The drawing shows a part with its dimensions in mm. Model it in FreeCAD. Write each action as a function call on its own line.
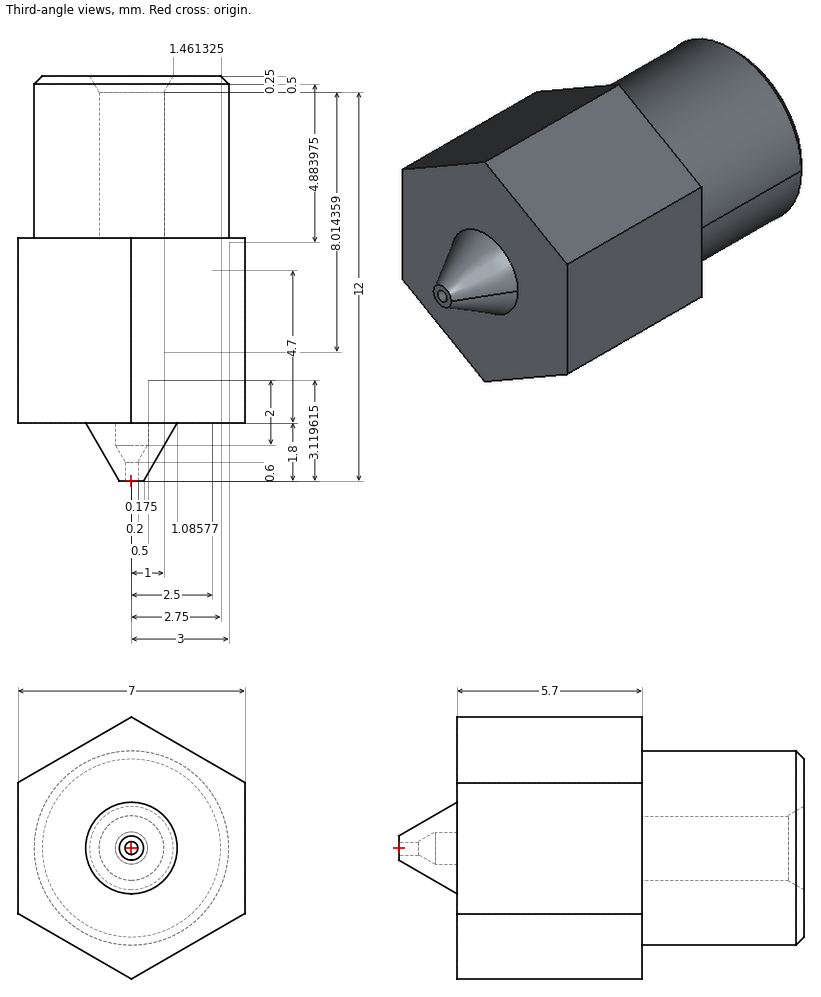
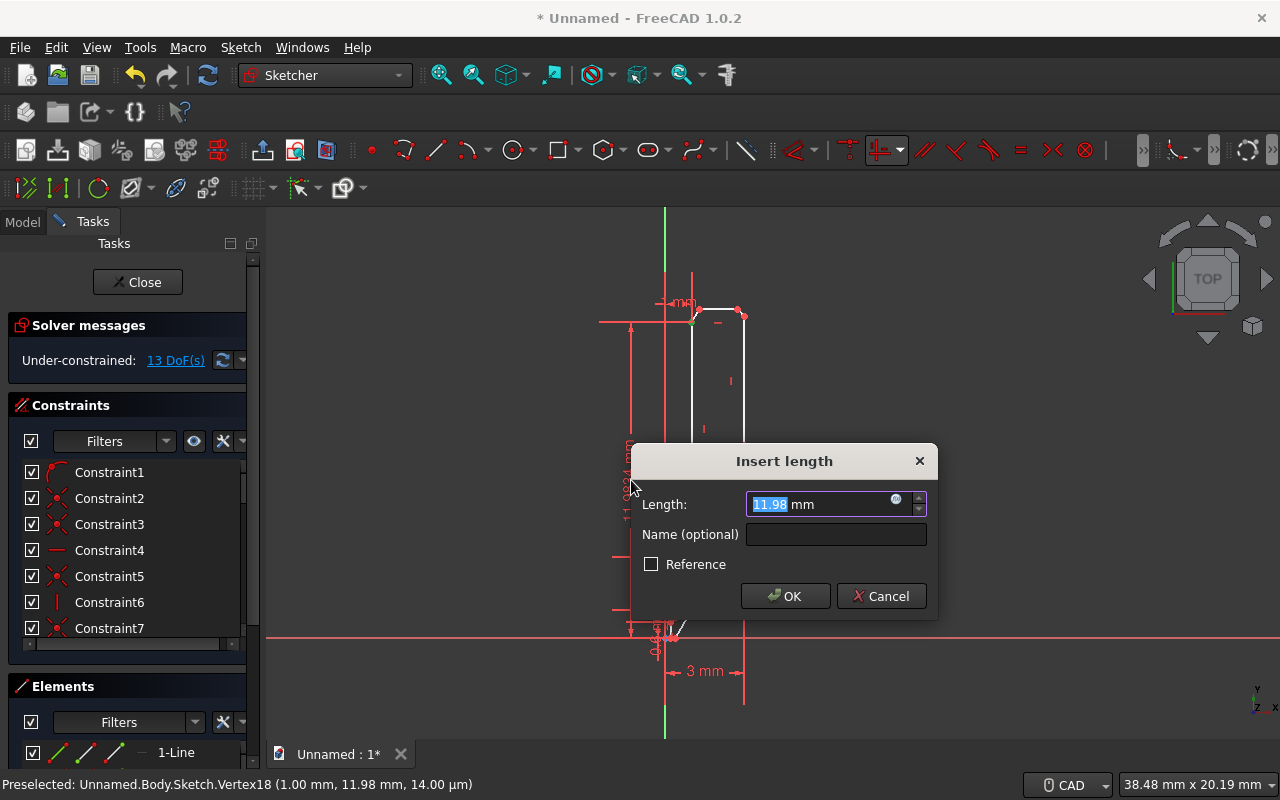
text(12)
key(Return)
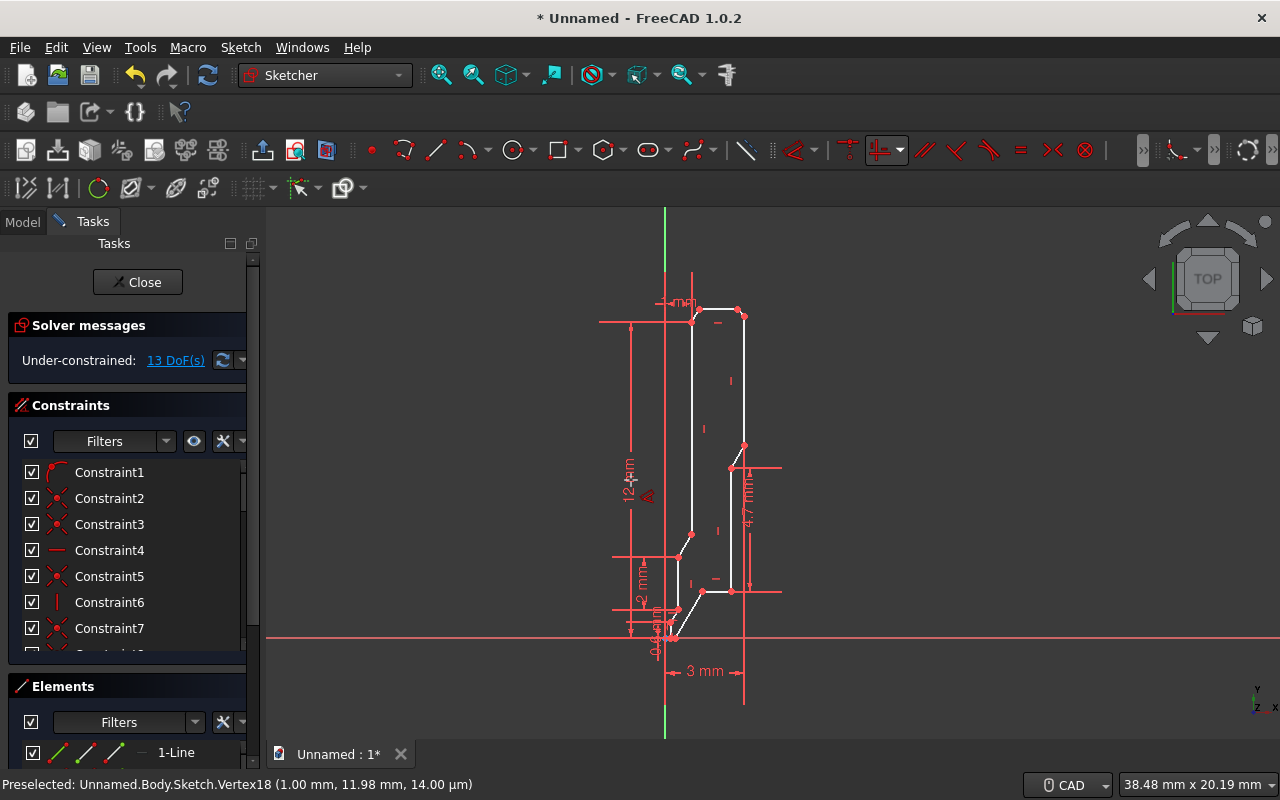
scroll(671, 638, up, 11)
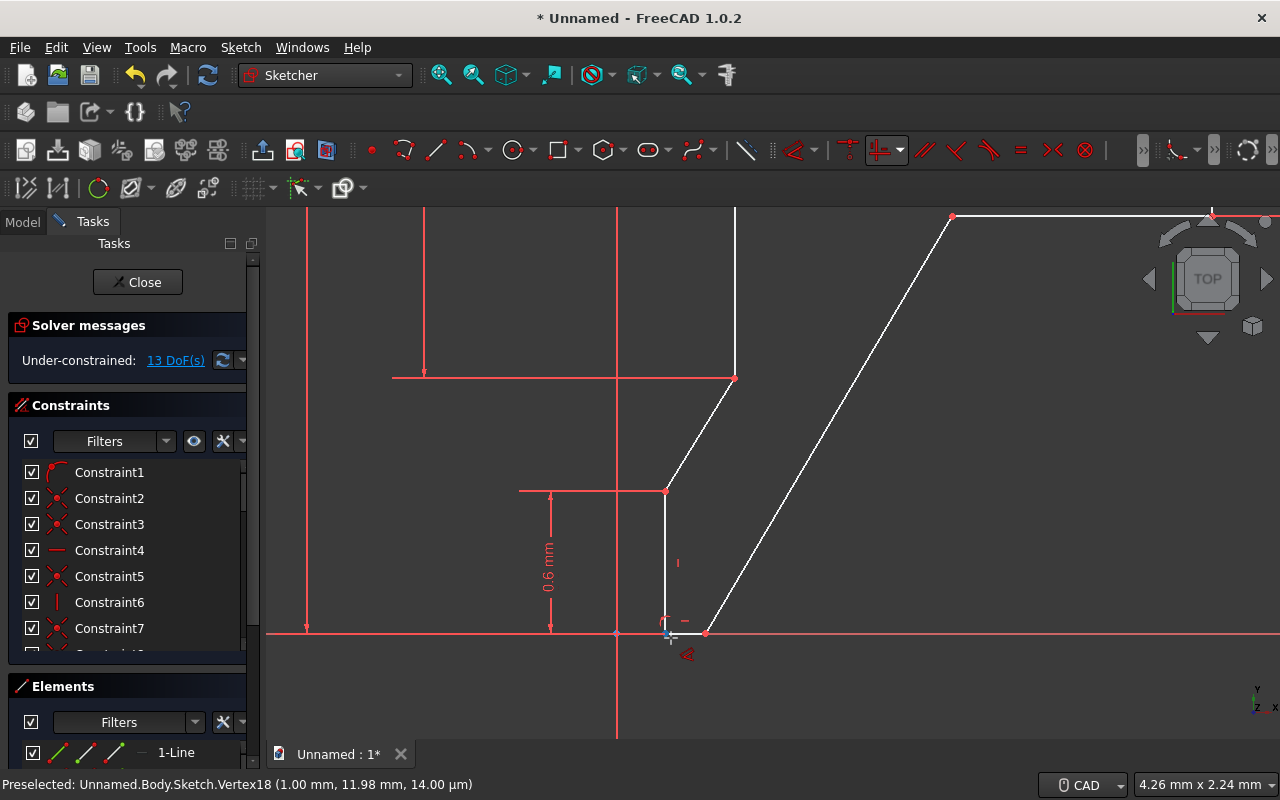
click(665, 634)
click(641, 668)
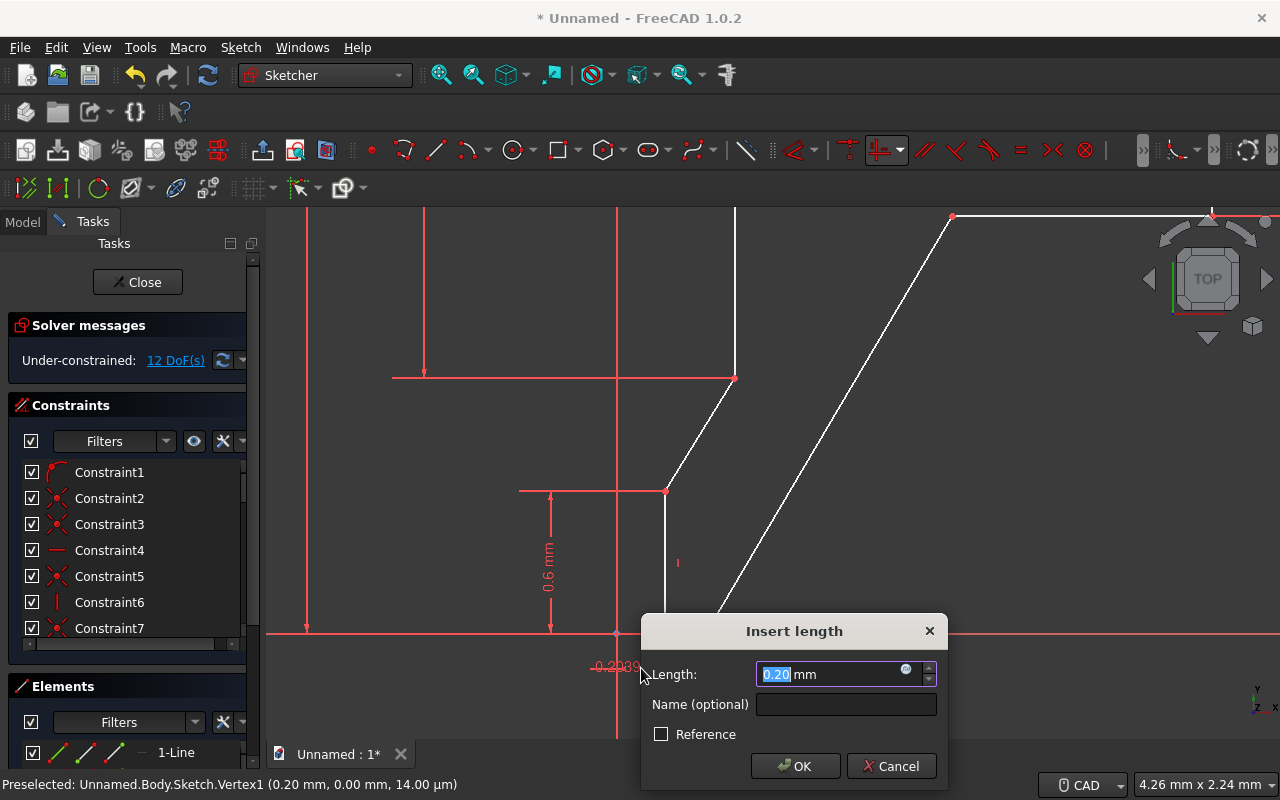
text(0.2)
key(Return)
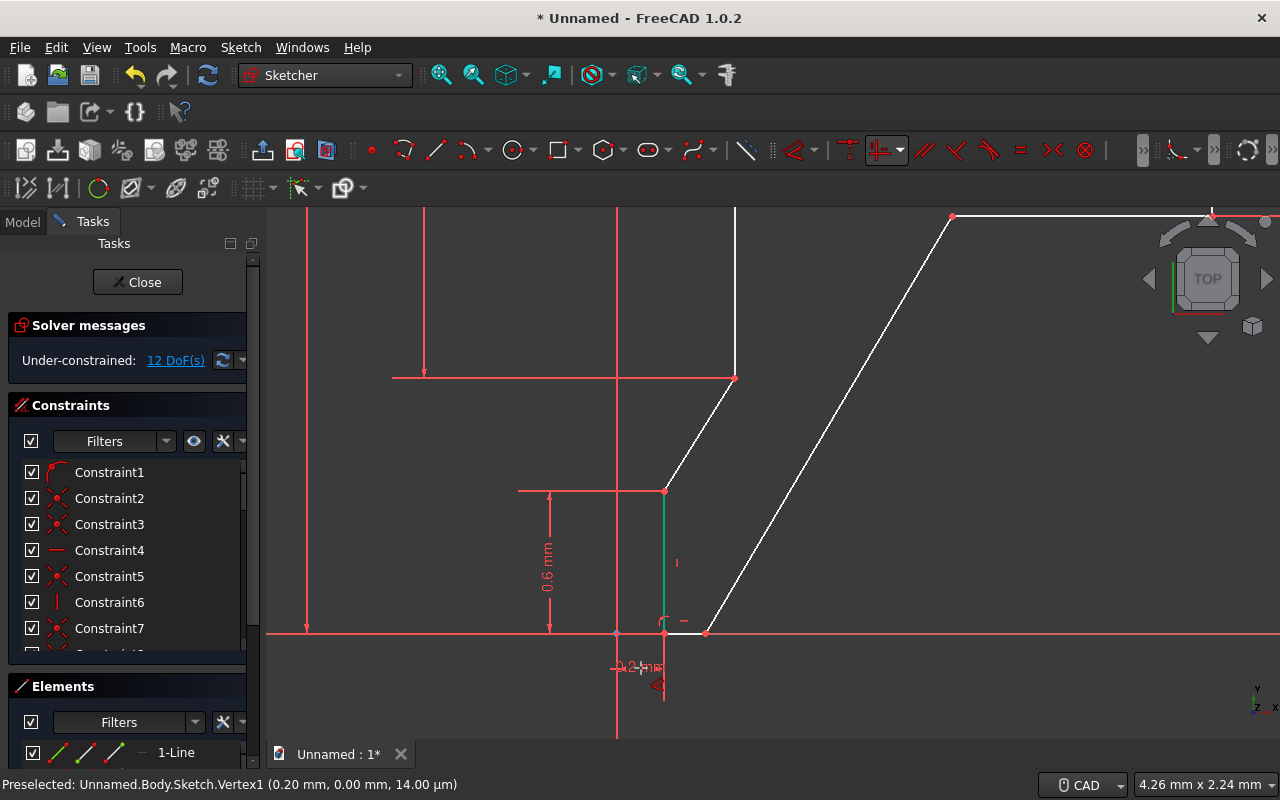
scroll(671, 638, down, 11)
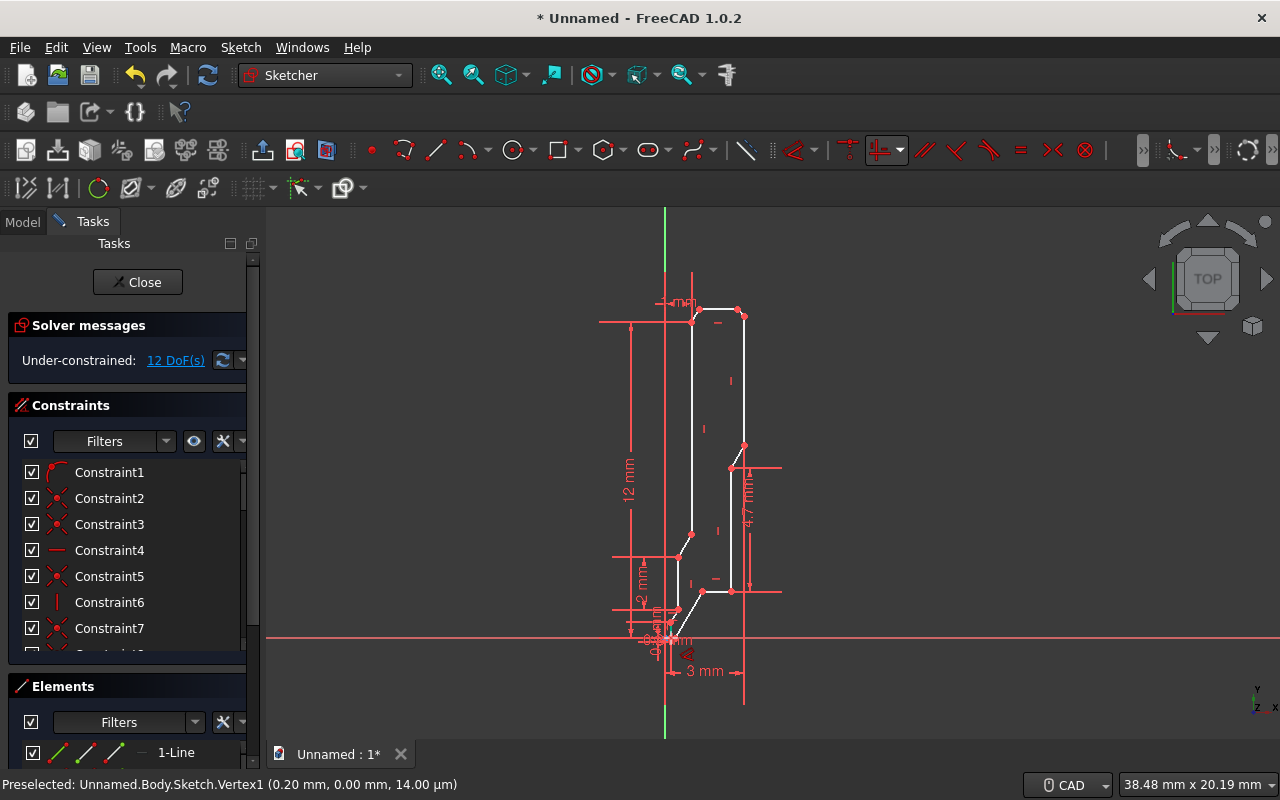
click(703, 592)
click(631, 604)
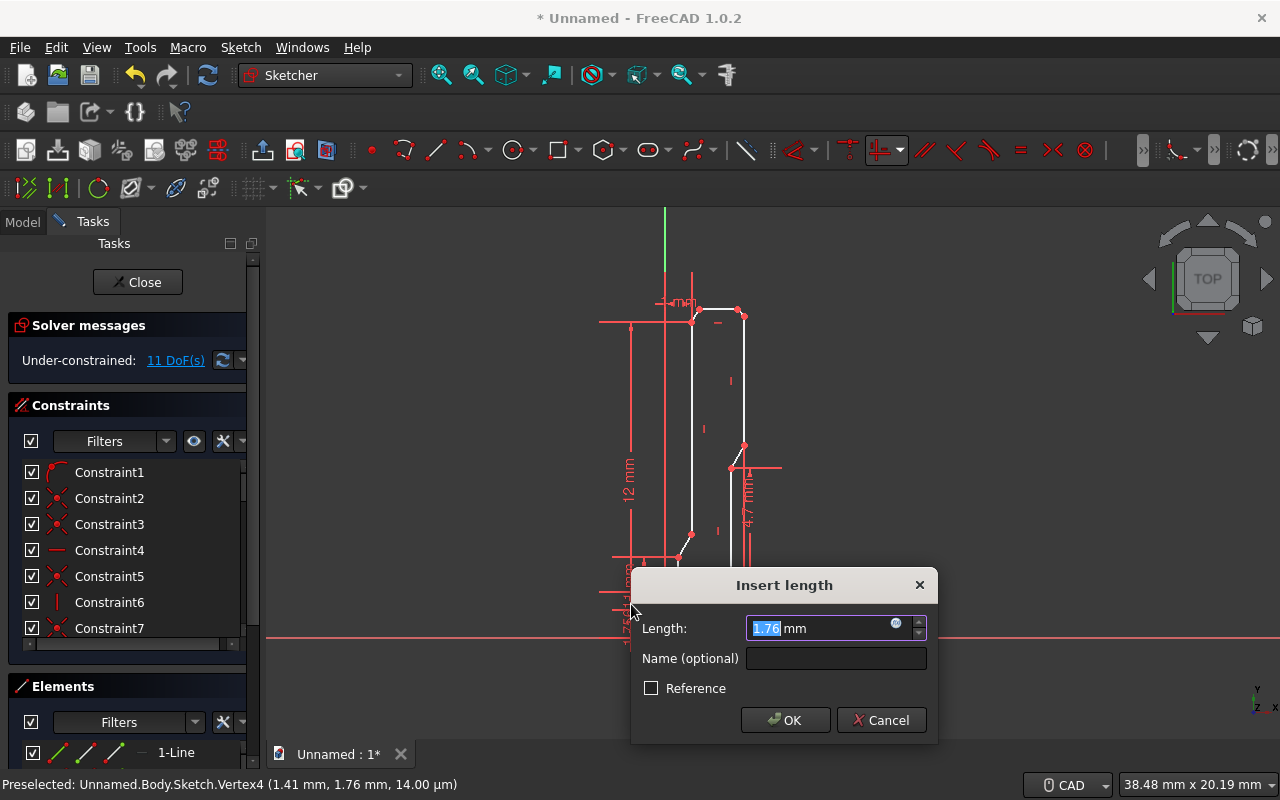
text(1.8)
key(Return)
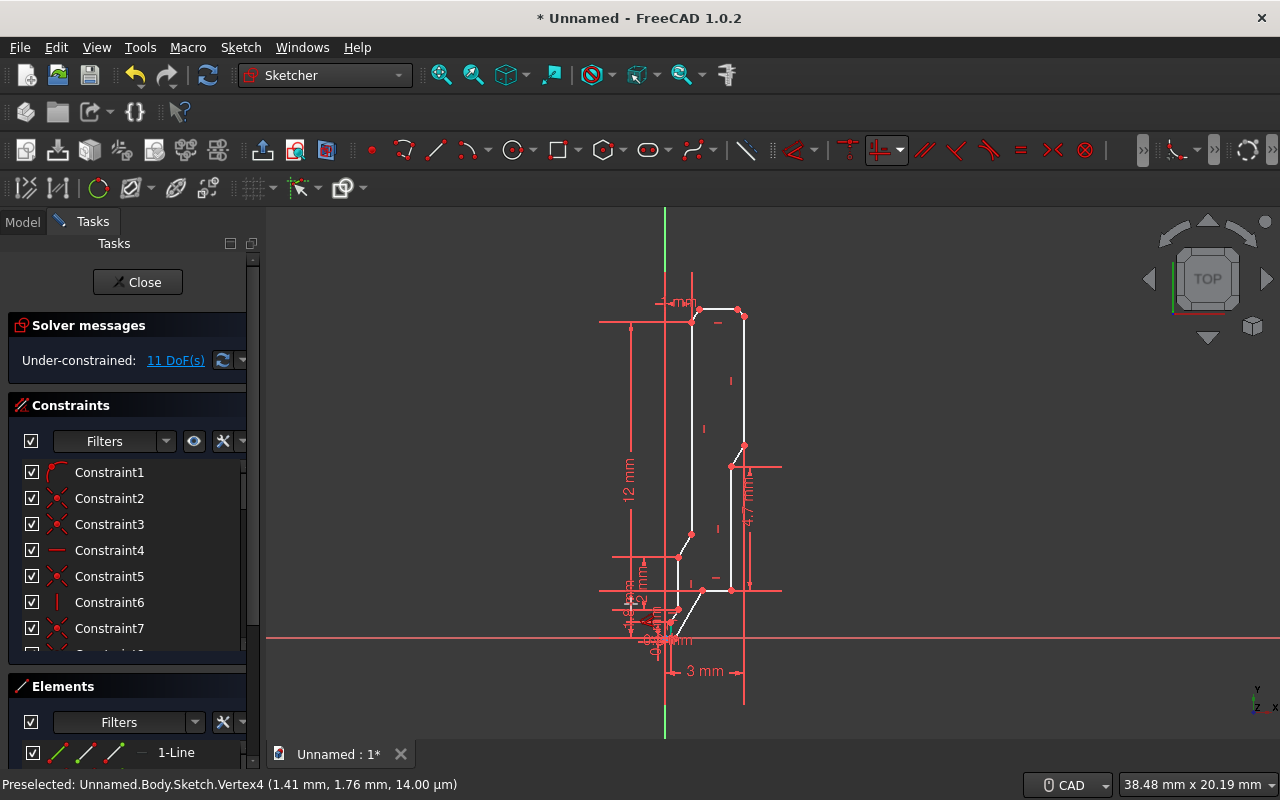
click(731, 591)
click(698, 557)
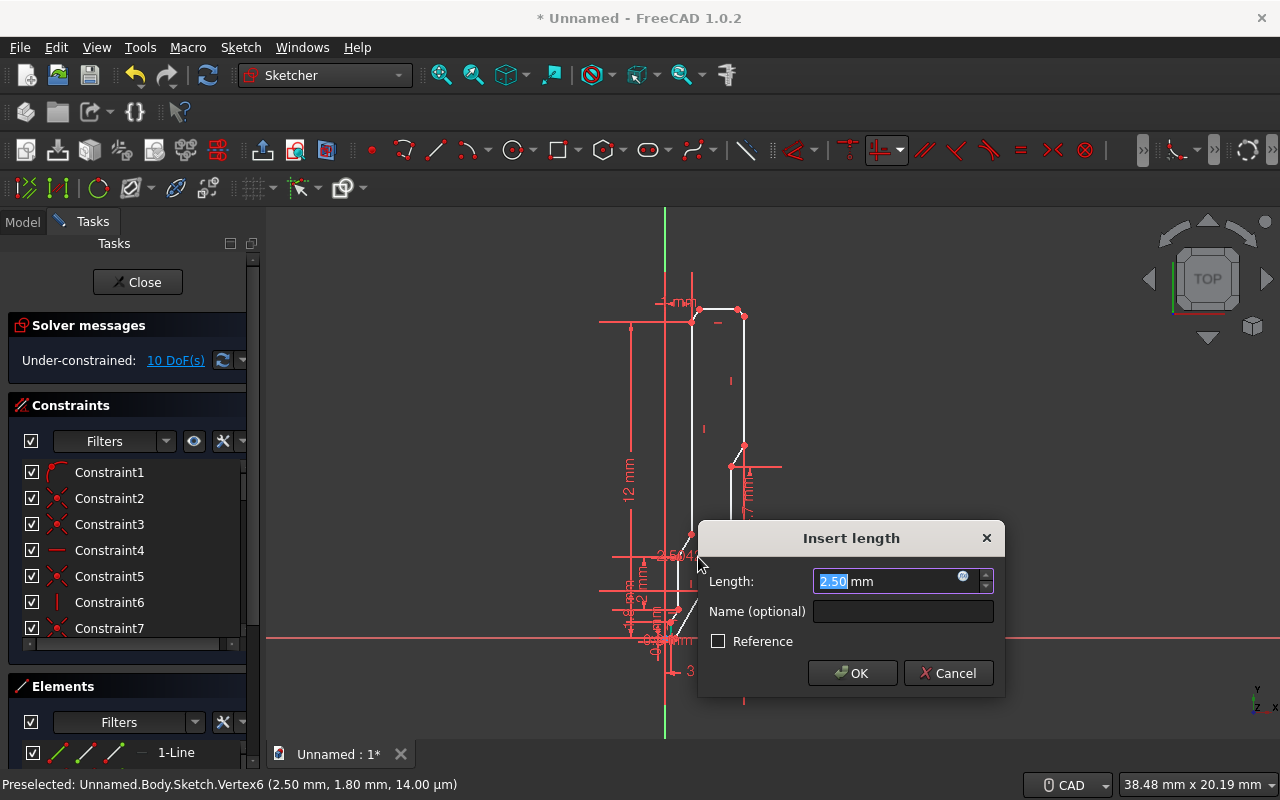
text(2.5)
key(Return)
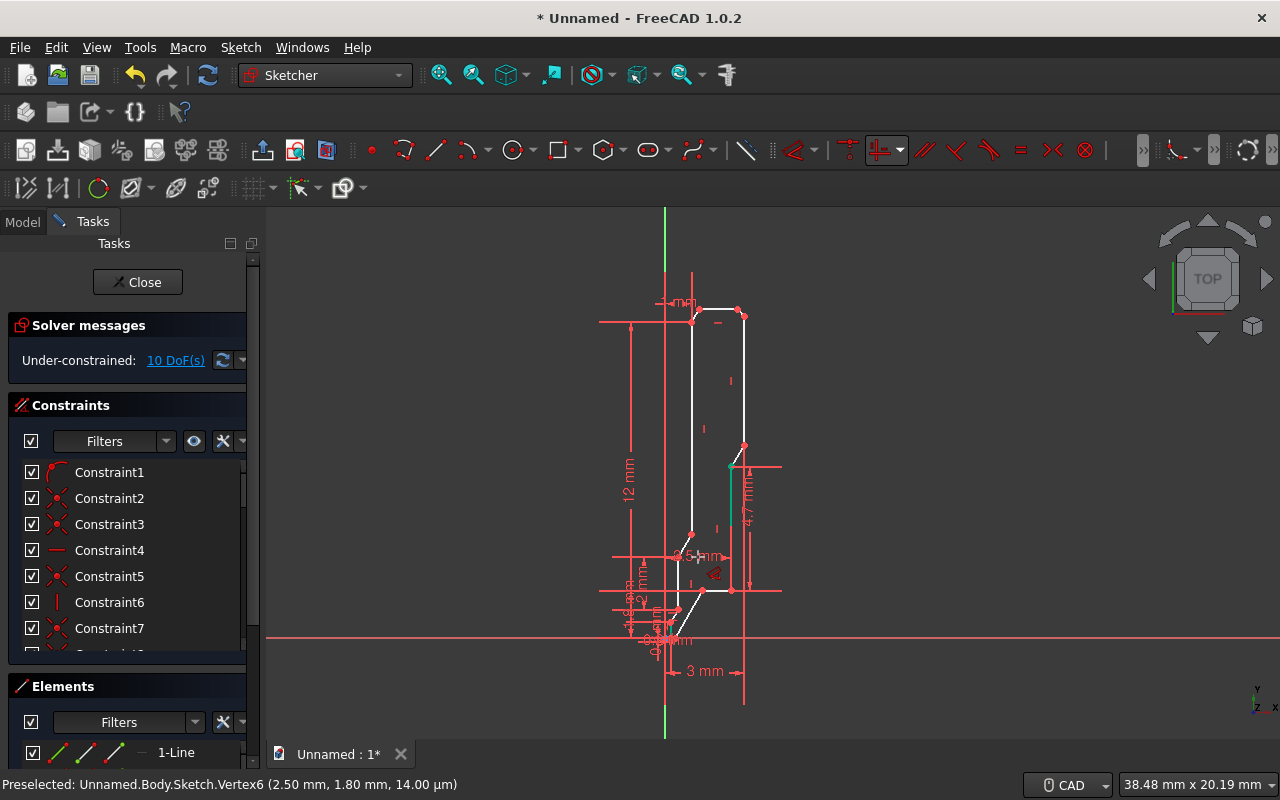
scroll(678, 557, up, 6)